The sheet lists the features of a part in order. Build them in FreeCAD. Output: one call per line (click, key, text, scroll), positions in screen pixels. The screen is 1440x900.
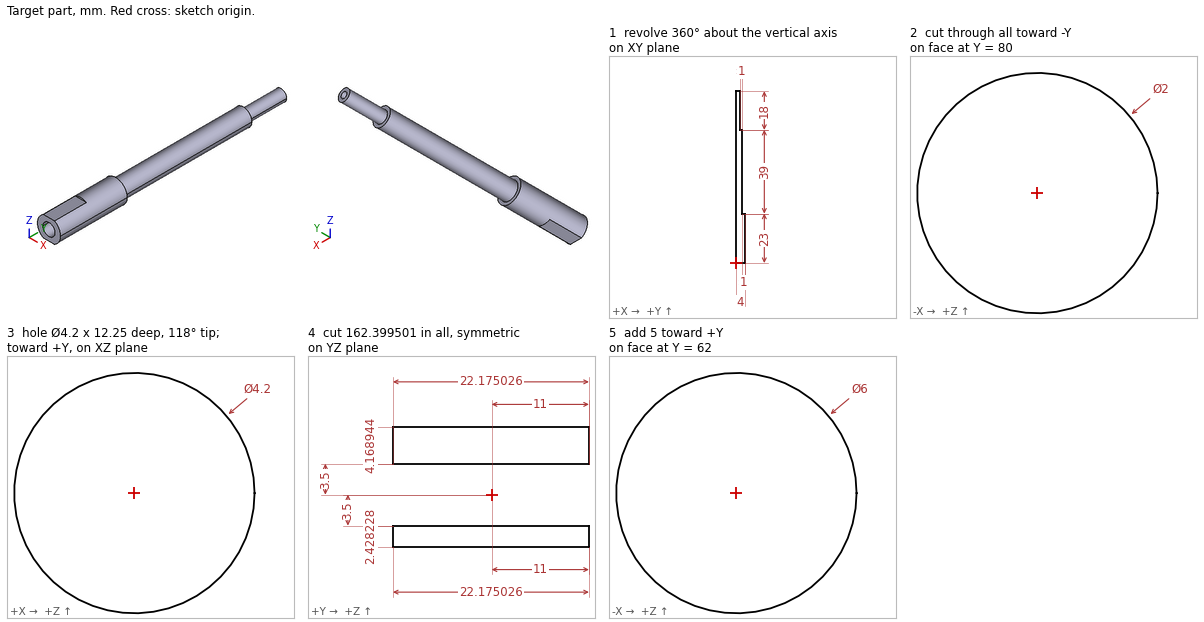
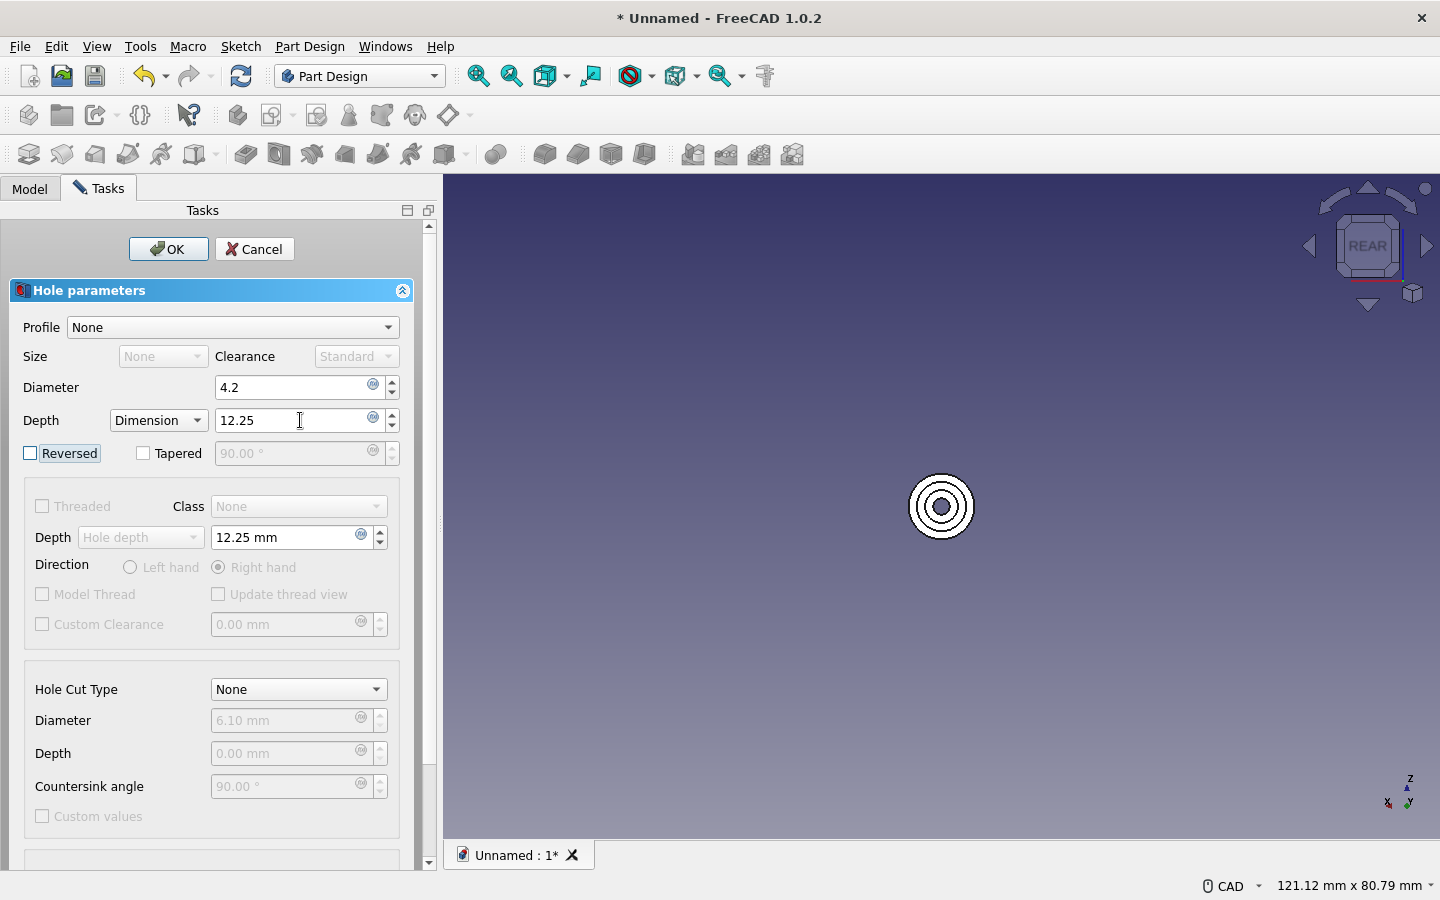
click(169, 249)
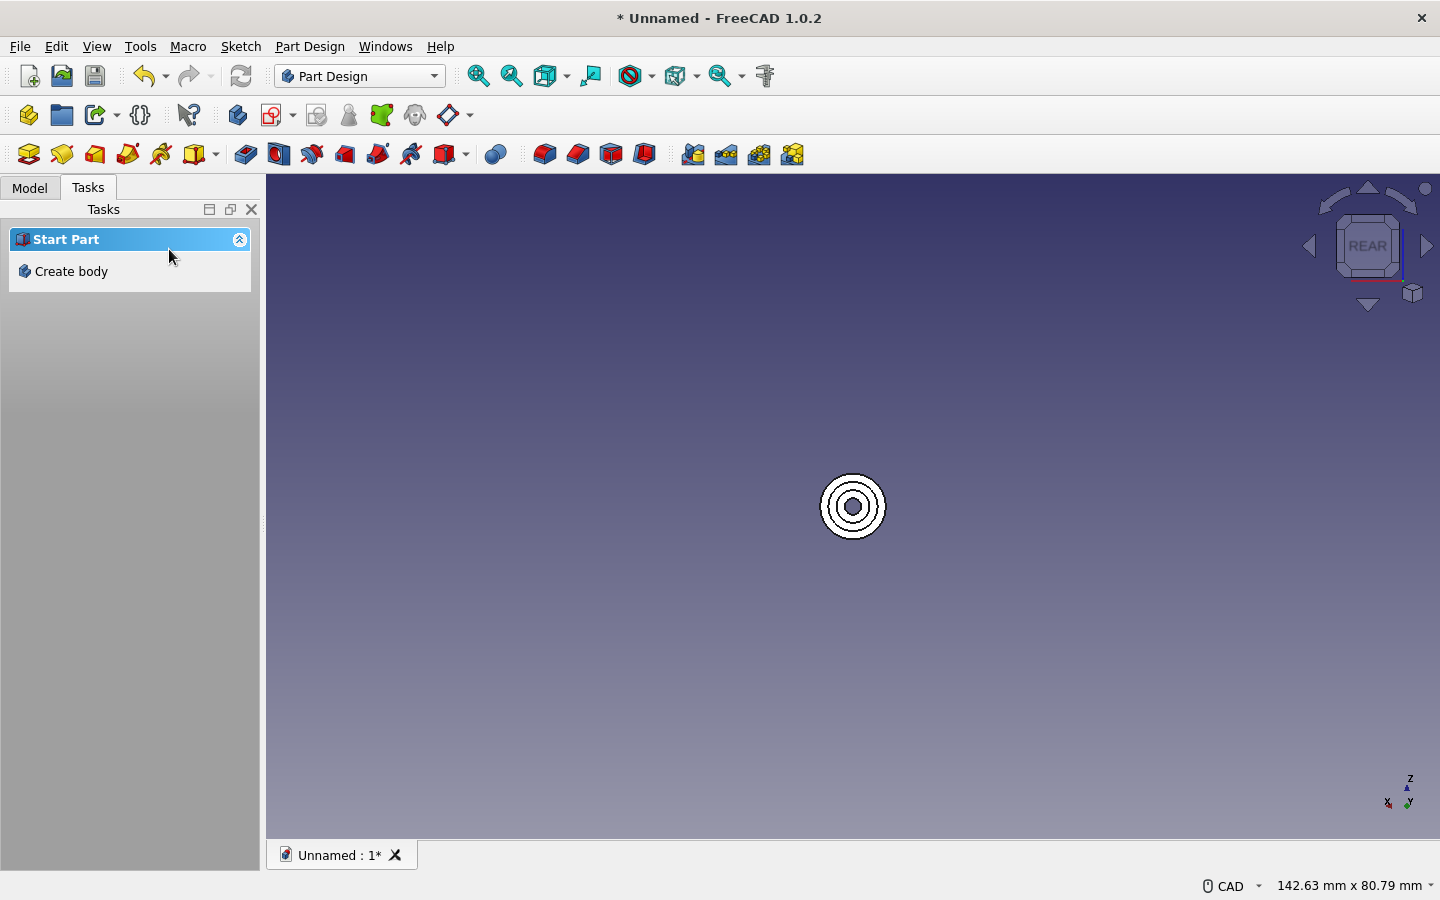
key(v)
key(f)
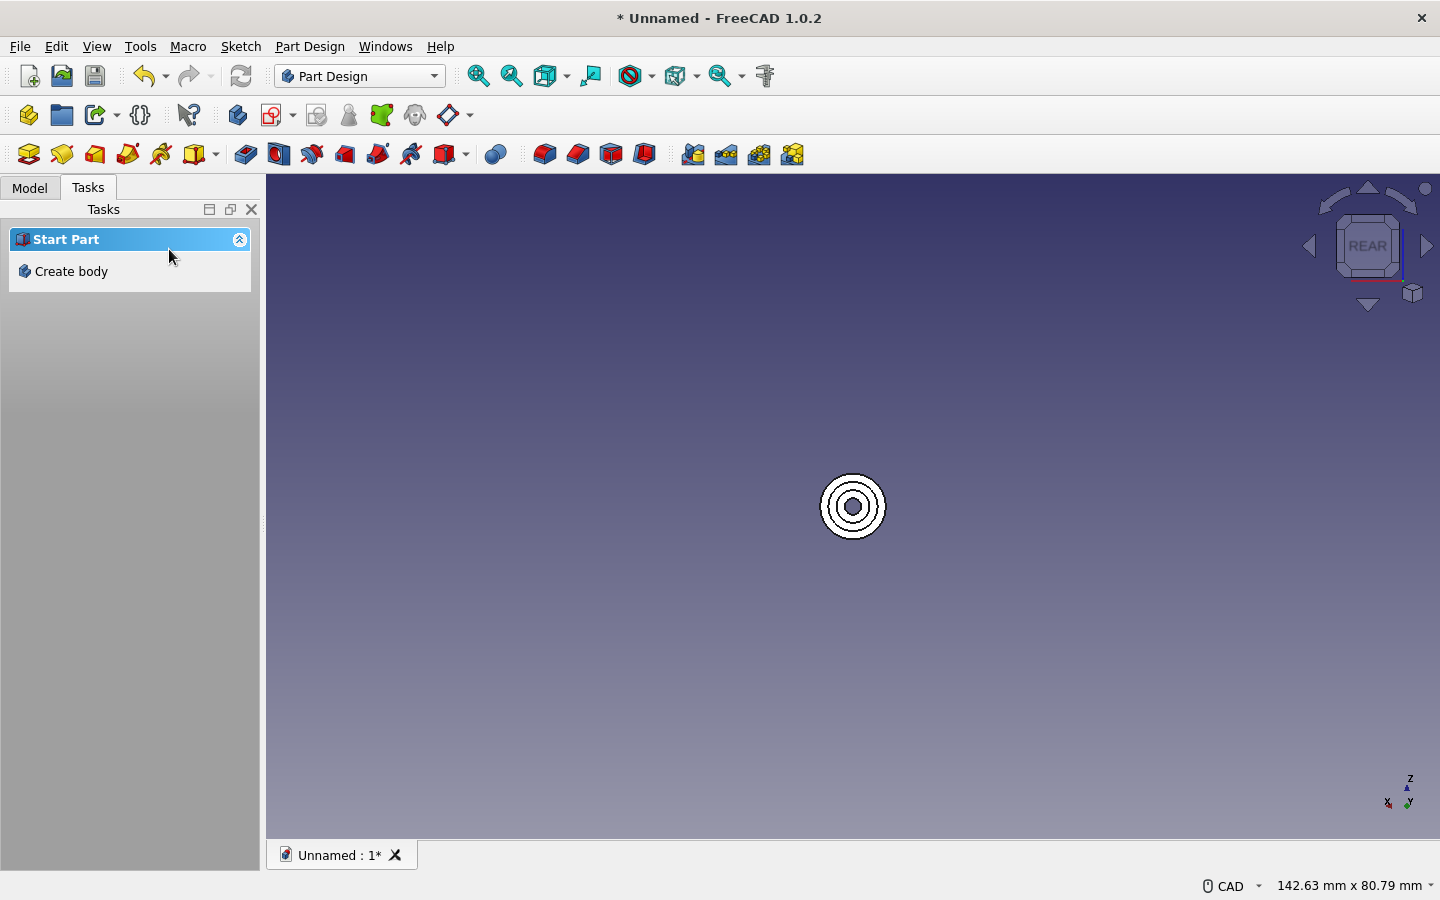
click(270, 116)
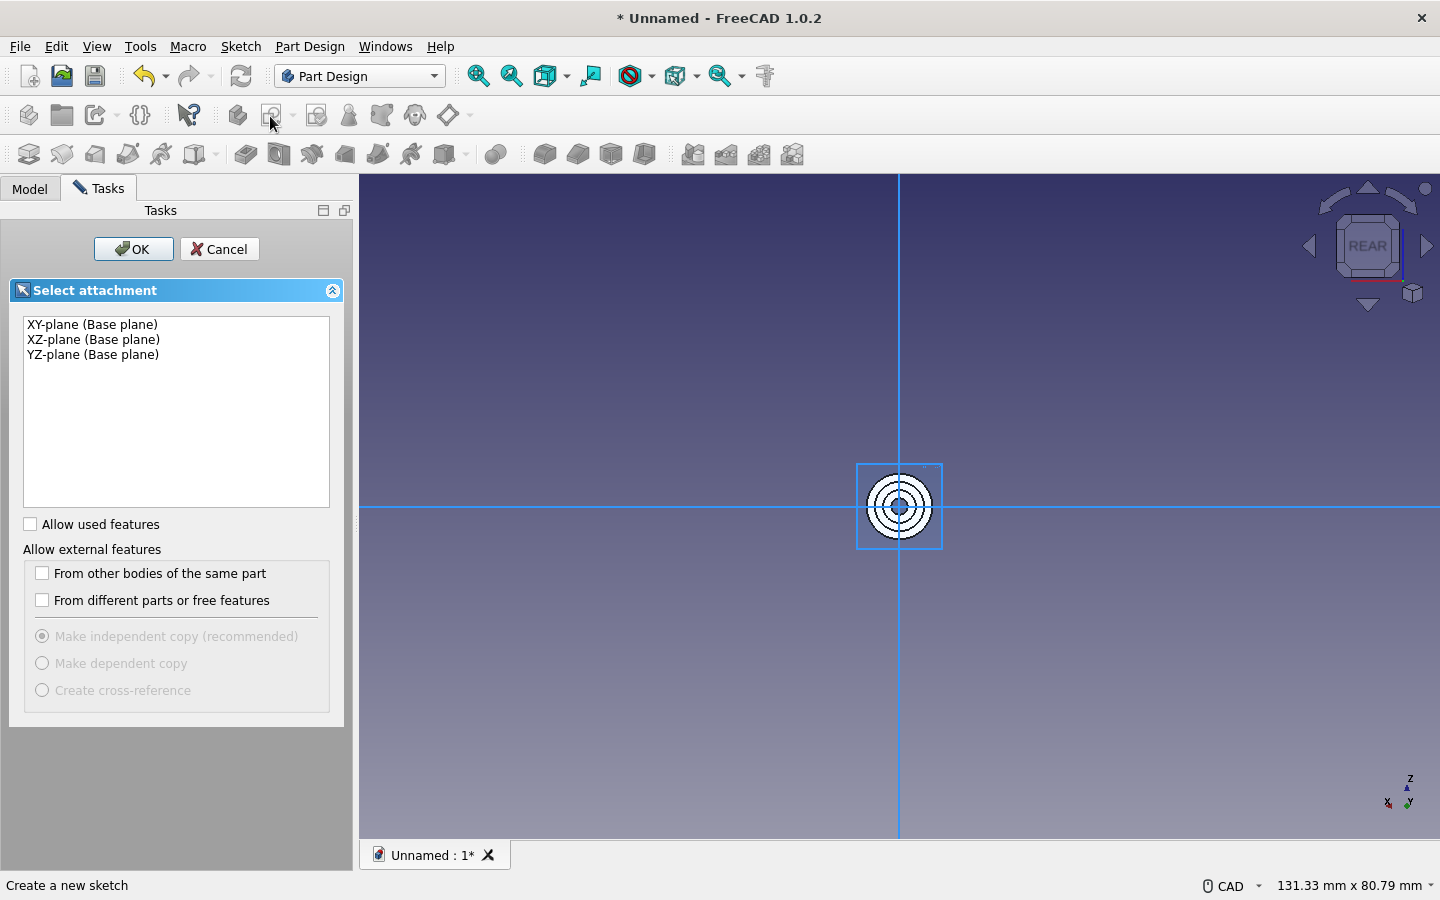
click(84, 354)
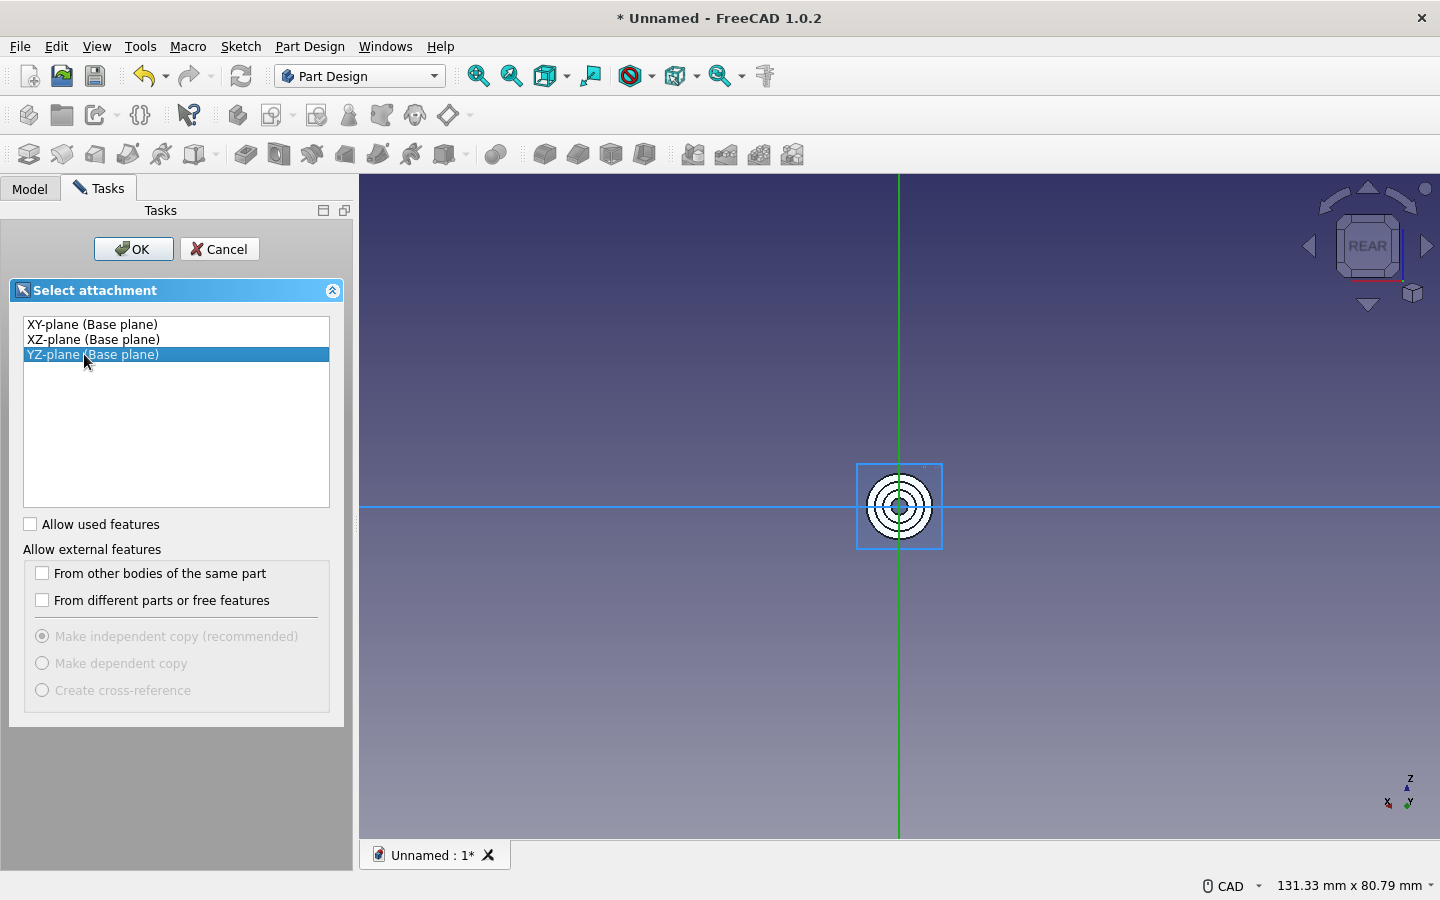
click(134, 249)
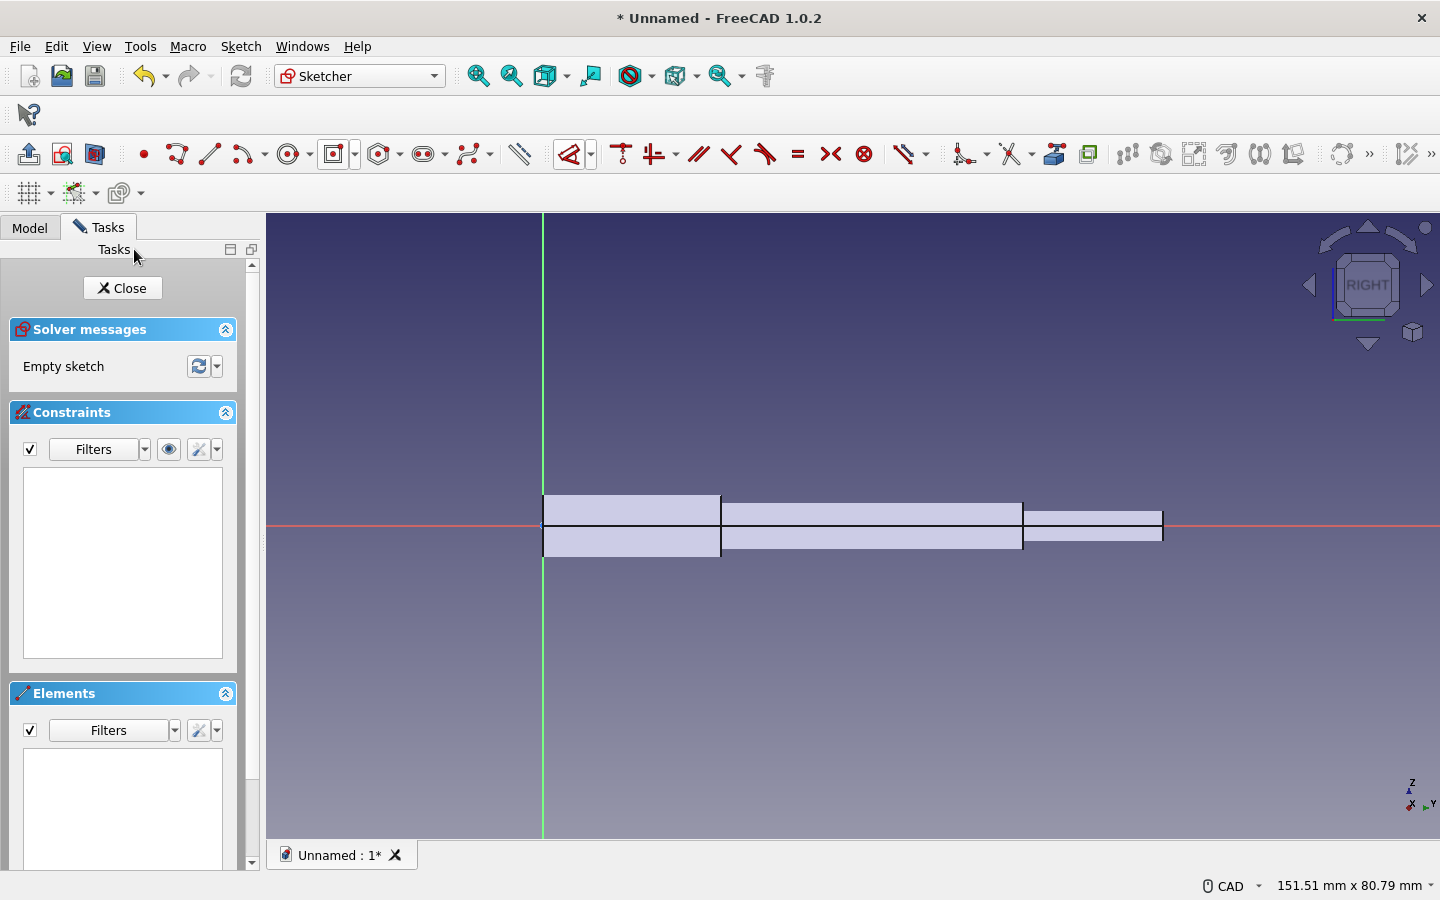
key(q)
key(s)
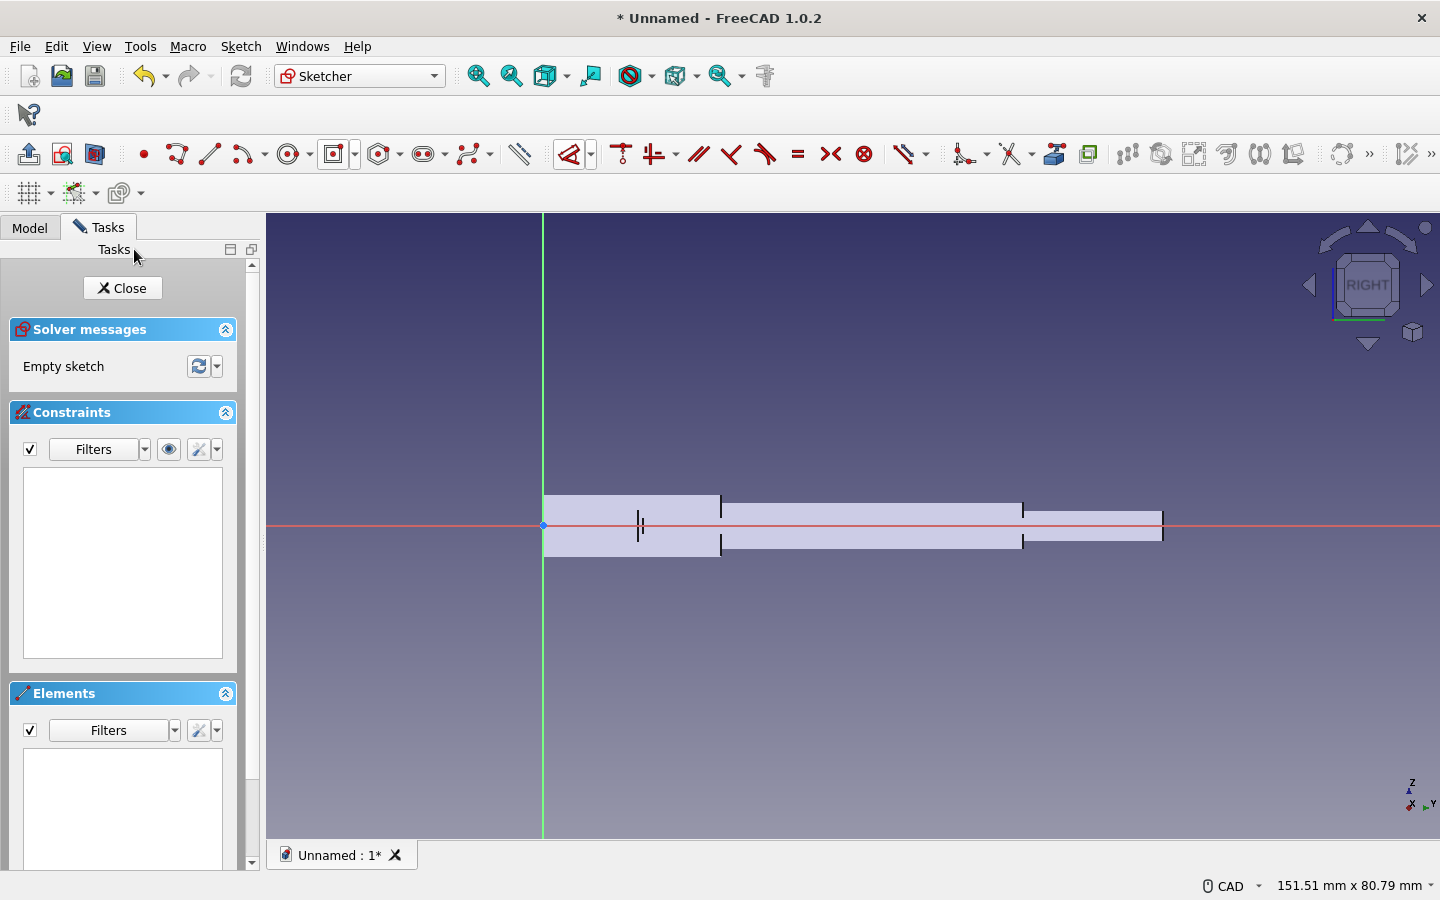
scroll(463, 517, up, 7)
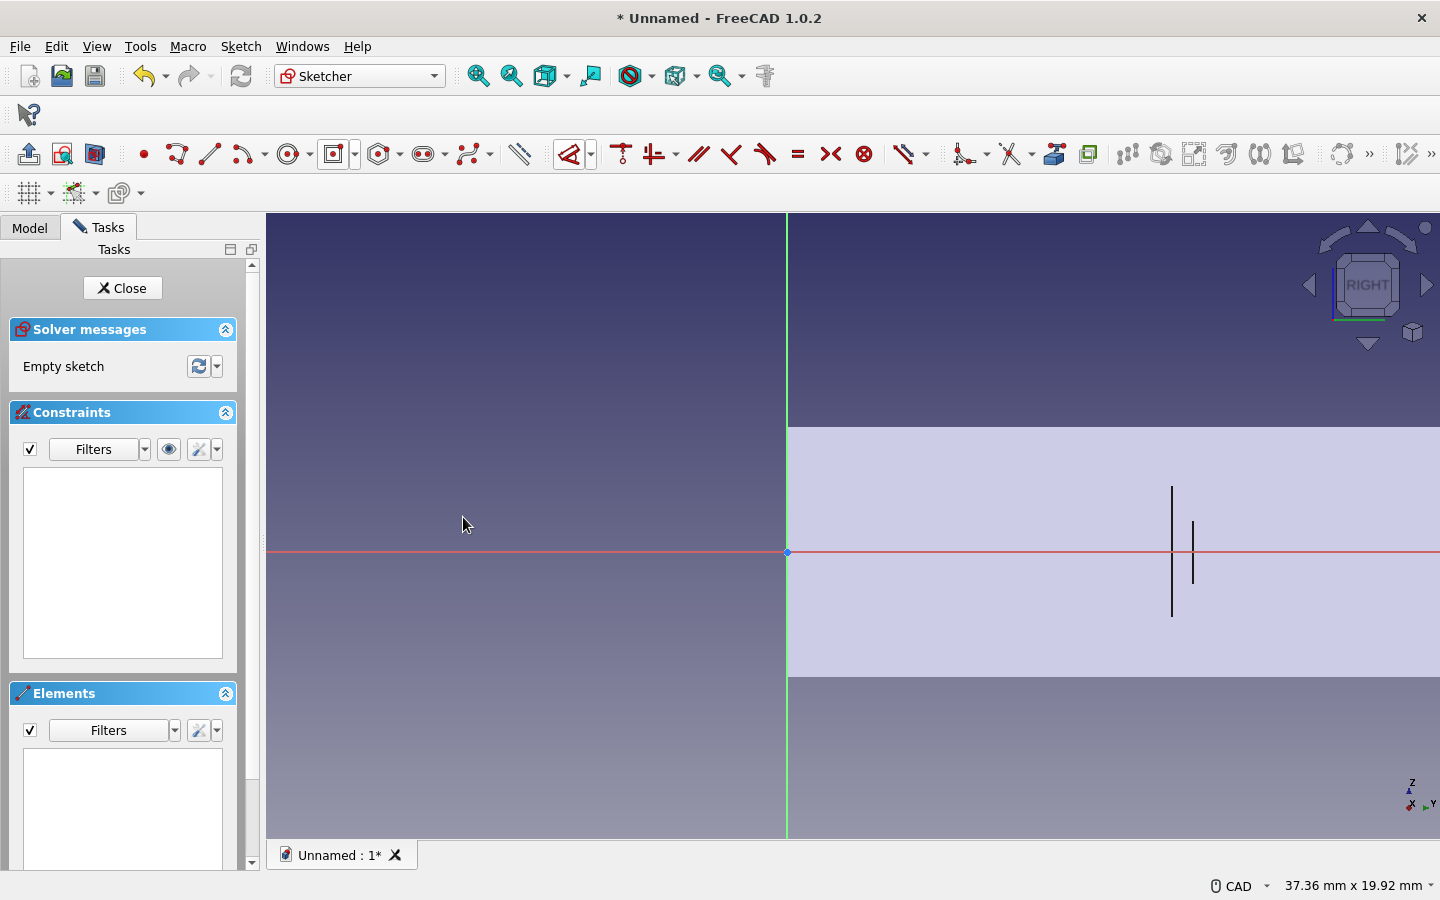
key(g)
key(r)